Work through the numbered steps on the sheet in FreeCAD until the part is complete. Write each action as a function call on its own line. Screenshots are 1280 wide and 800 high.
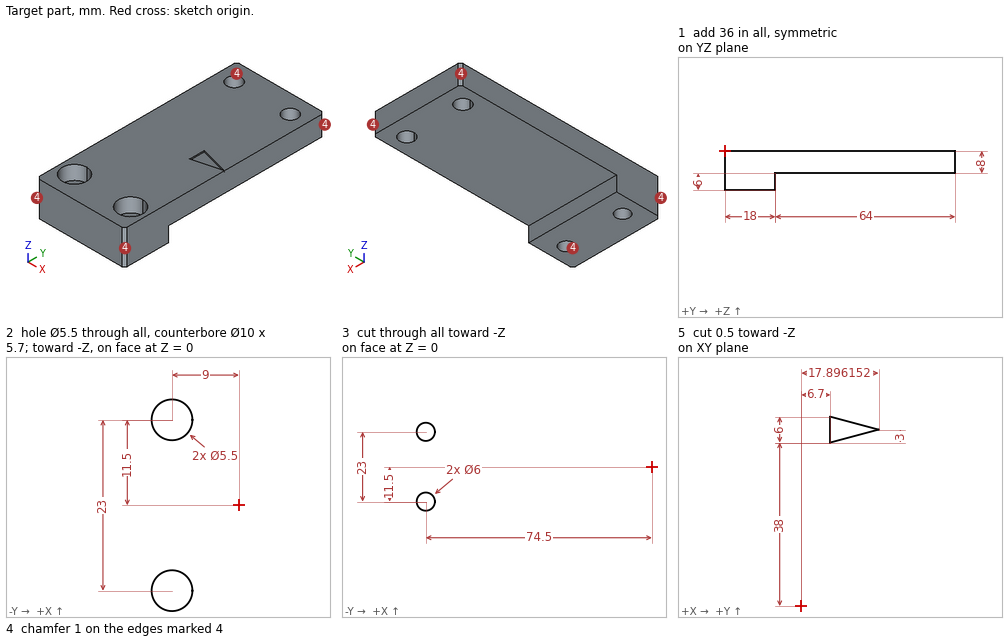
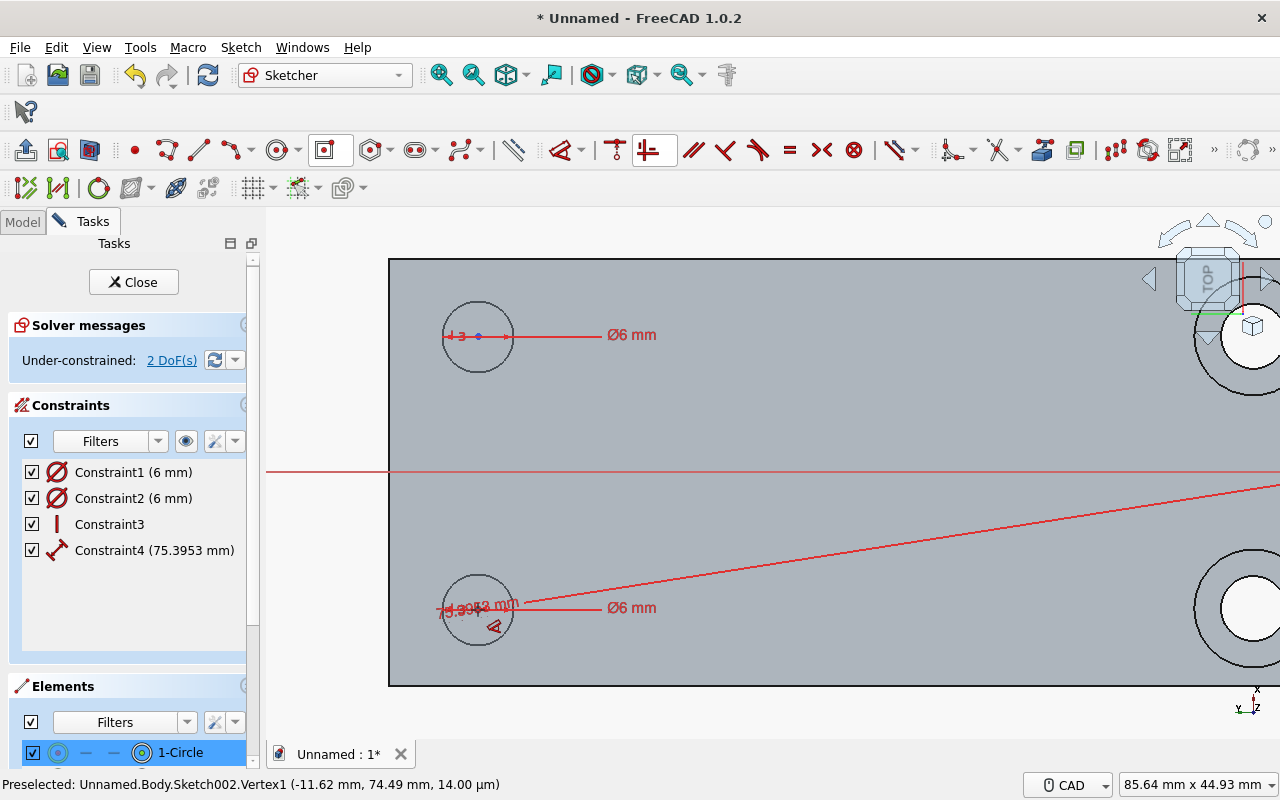
click(478, 337)
click(512, 411)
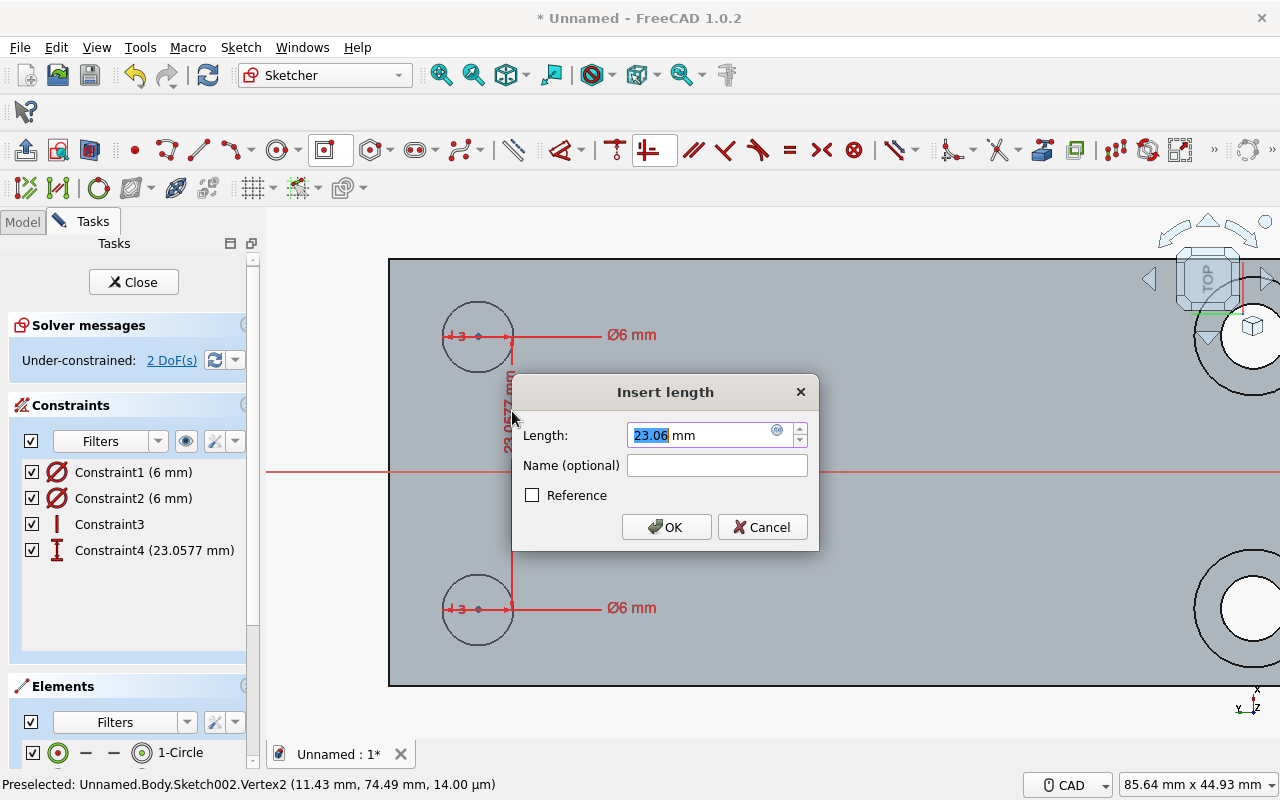
text(23)
key(Return)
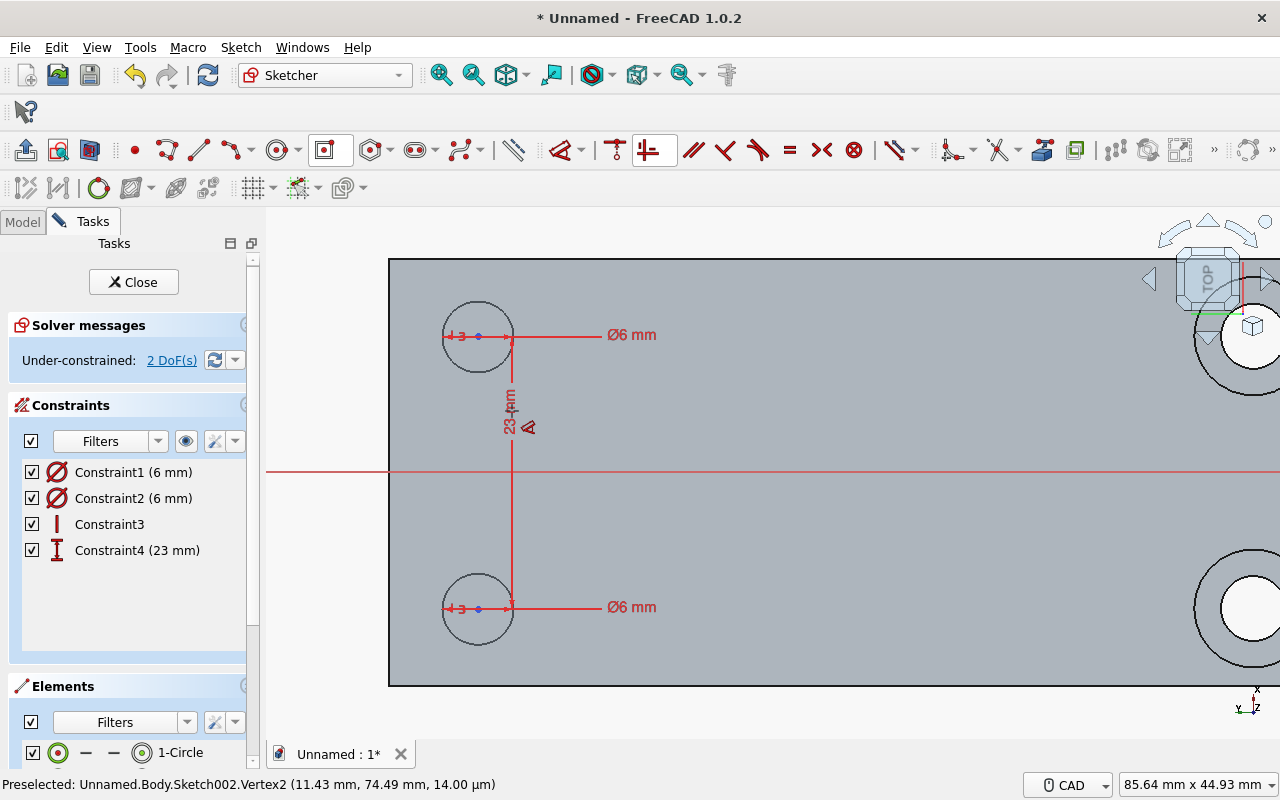
click(478, 609)
click(796, 643)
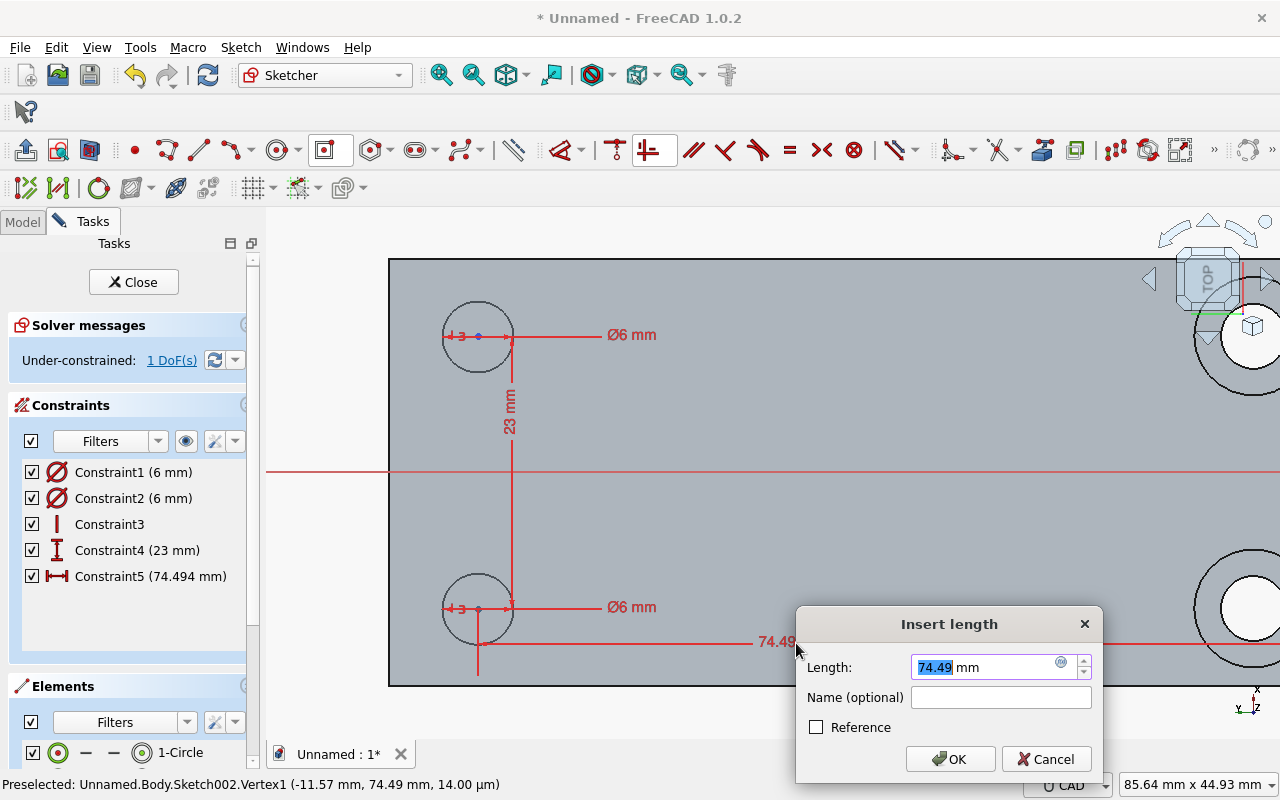
text(74.5)
key(Return)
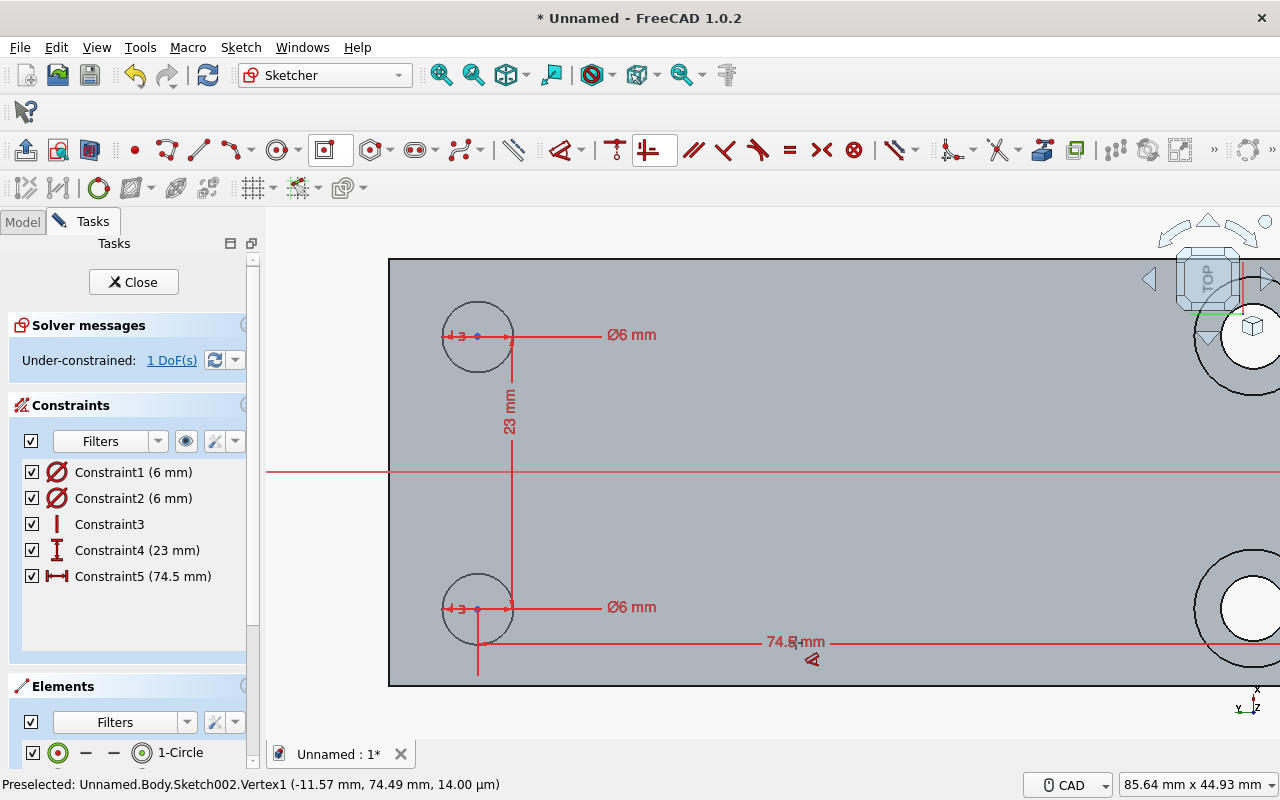
click(478, 609)
click(444, 541)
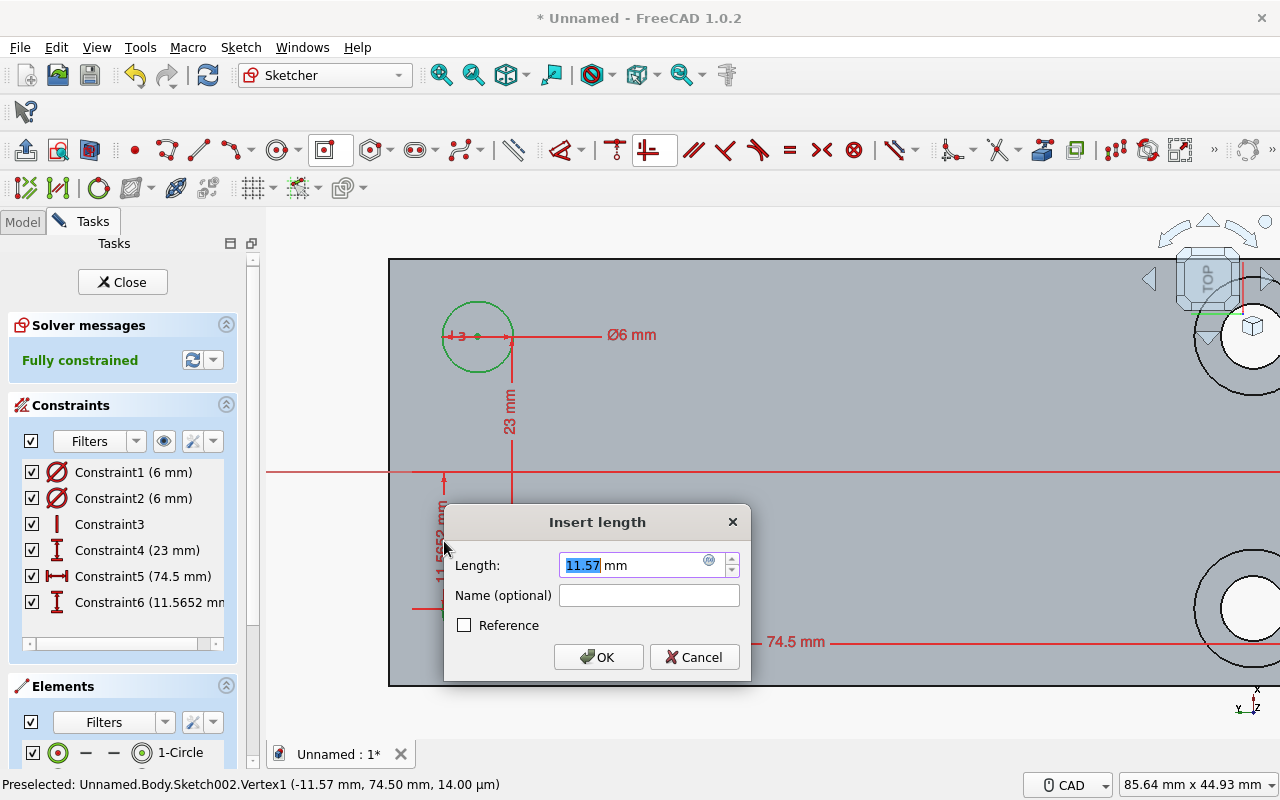
text(11.5)
key(Return)
key(Escape)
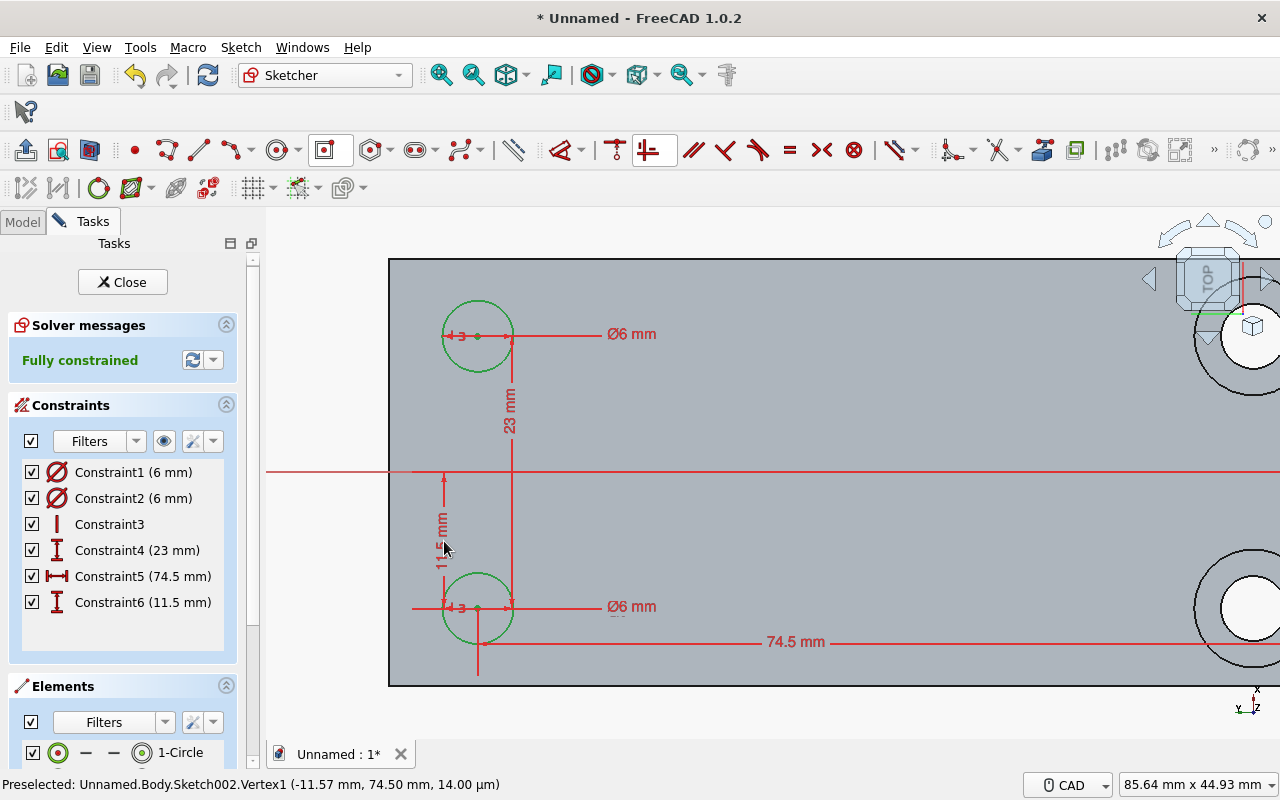
click(123, 282)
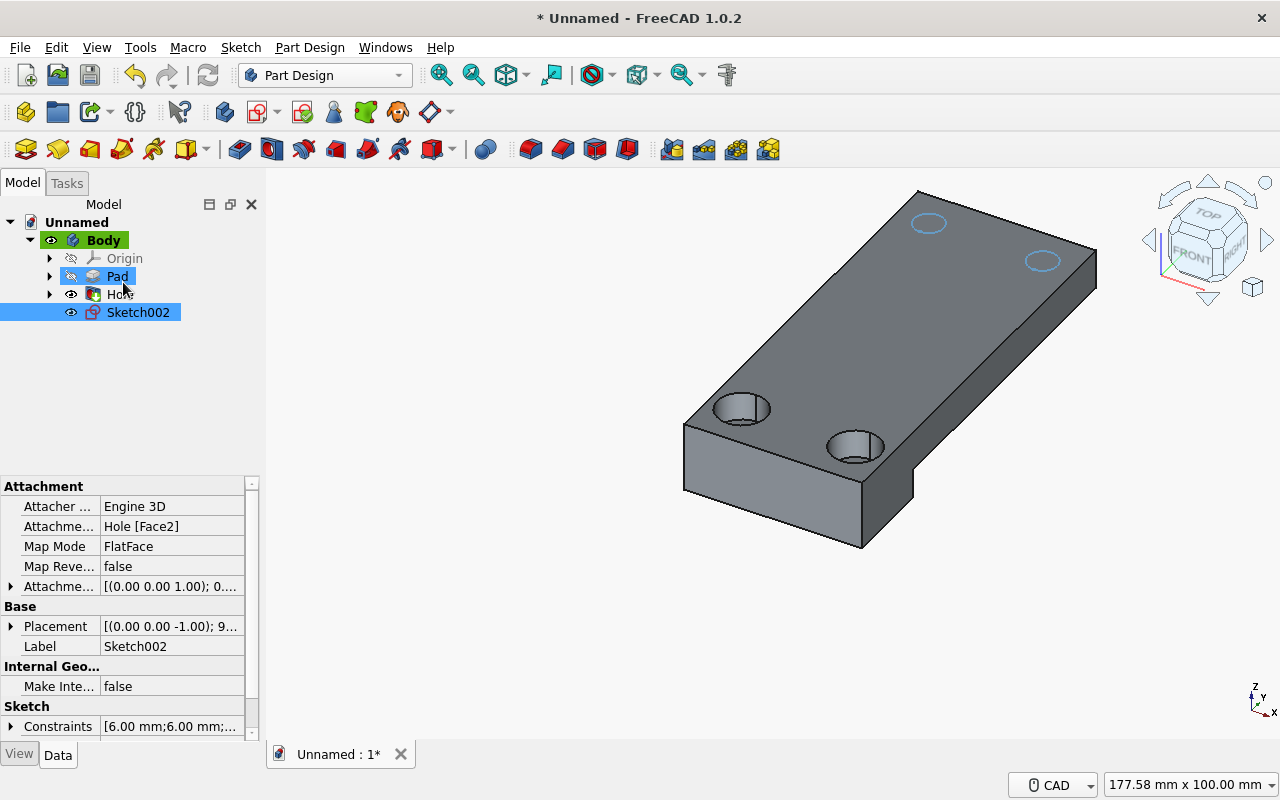
click(240, 150)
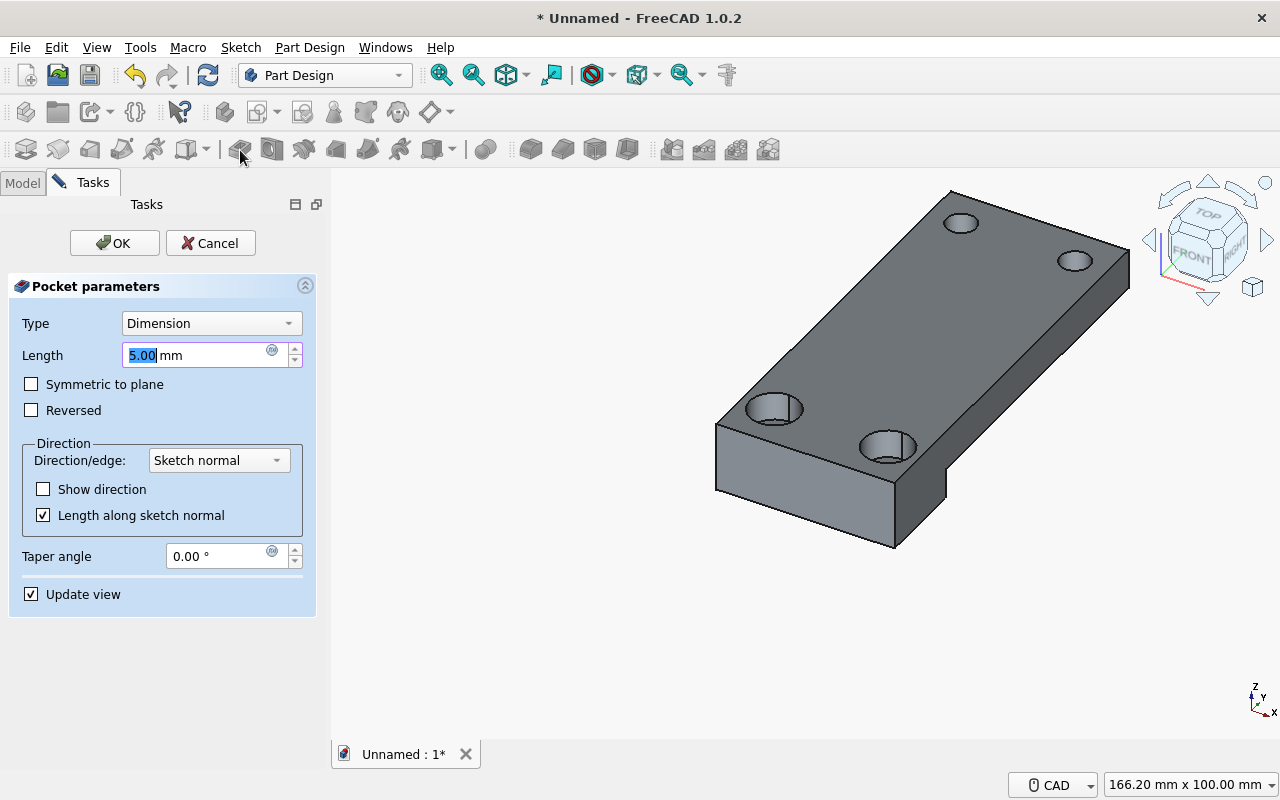
click(212, 324)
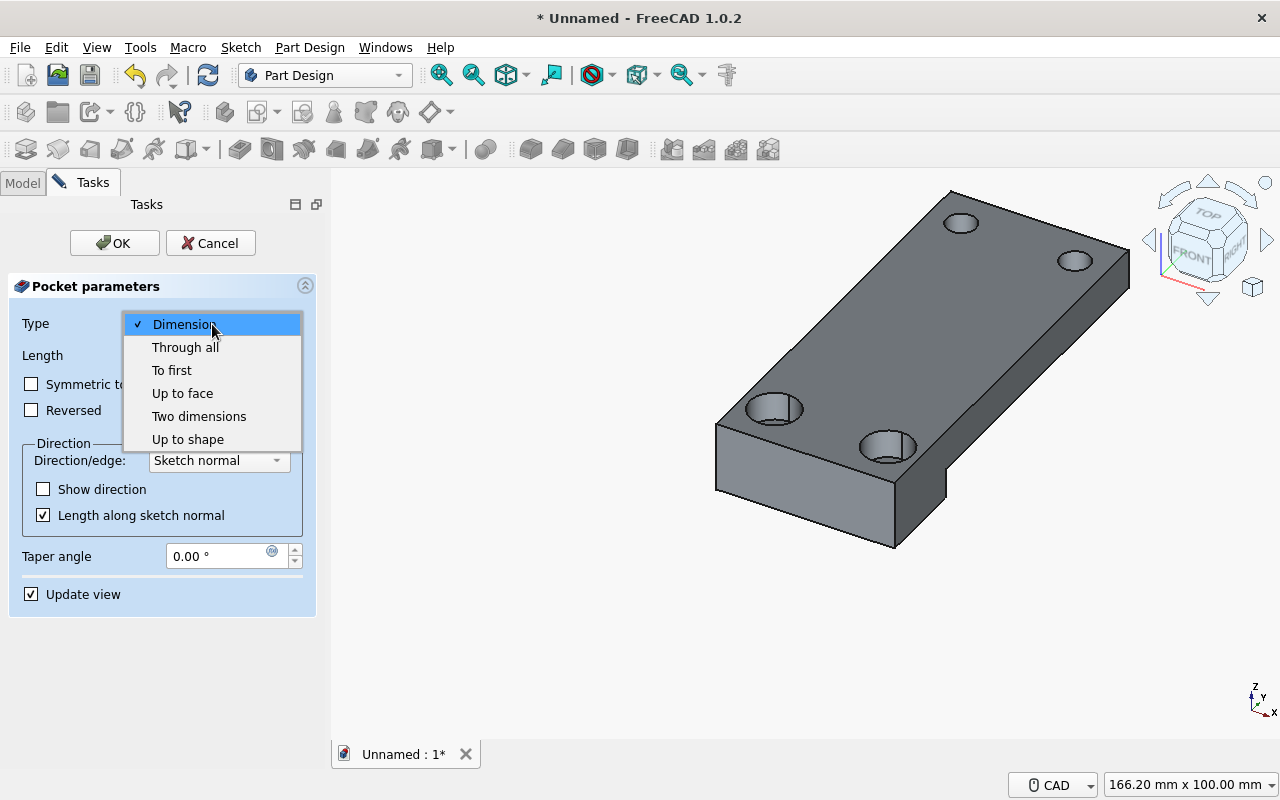
click(212, 348)